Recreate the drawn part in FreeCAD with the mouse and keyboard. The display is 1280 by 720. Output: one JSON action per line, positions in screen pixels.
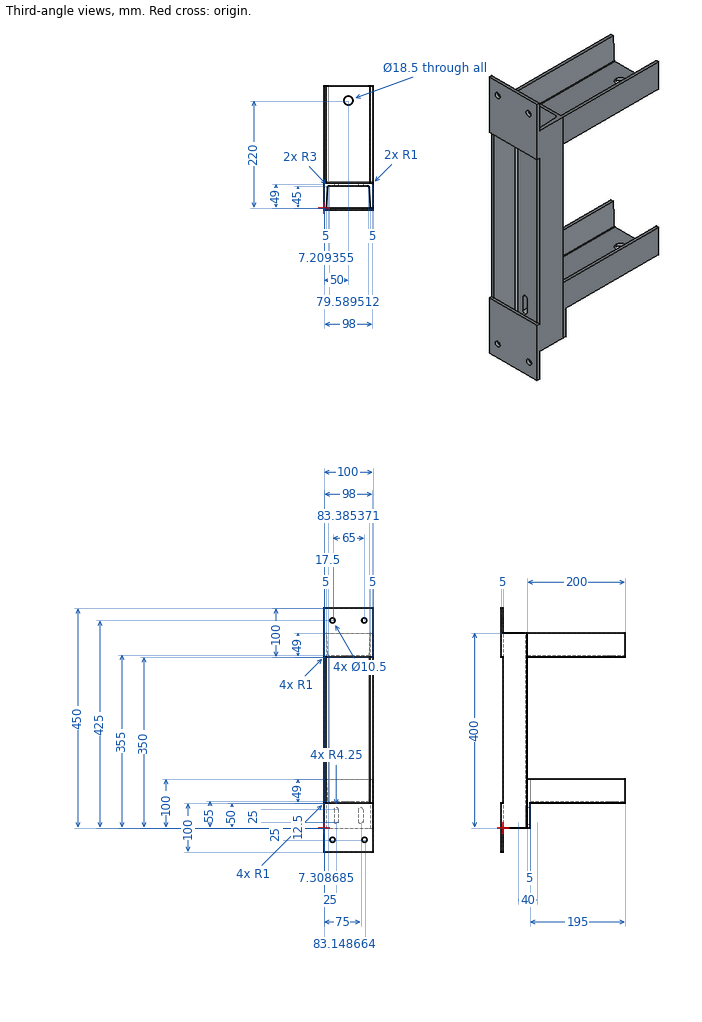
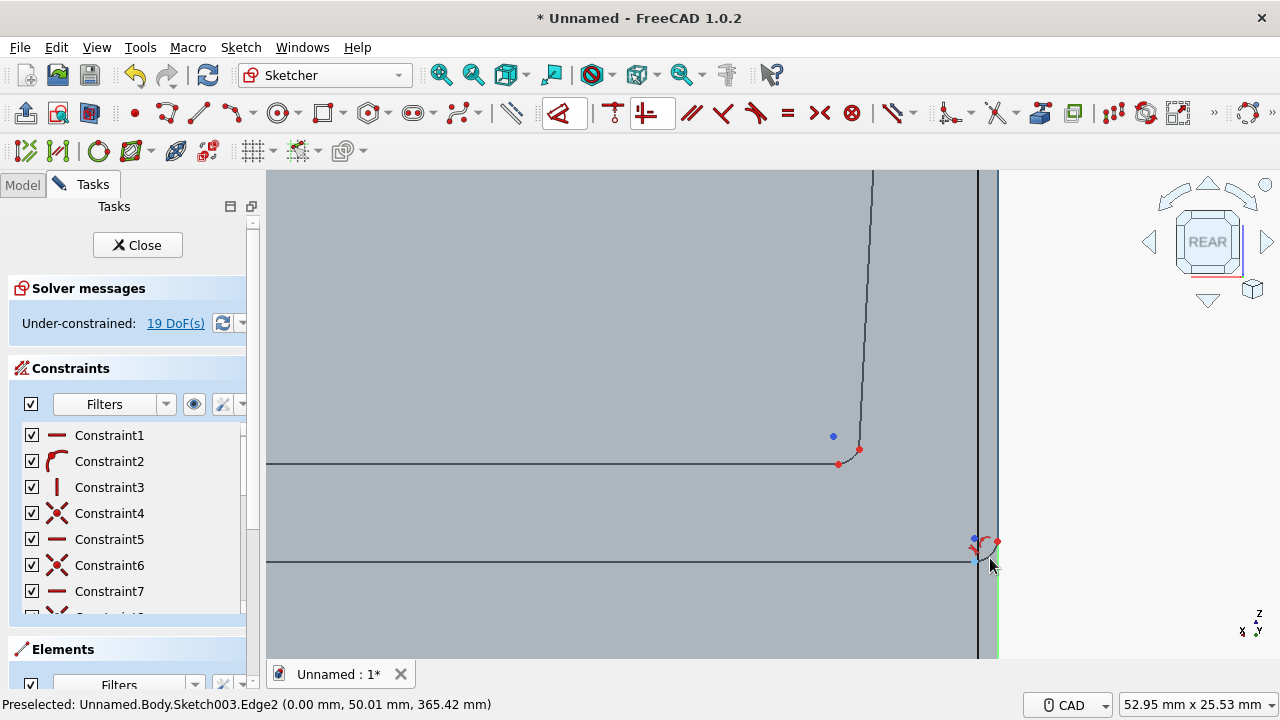
{"action": "left_click", "coordinate": [990, 556]}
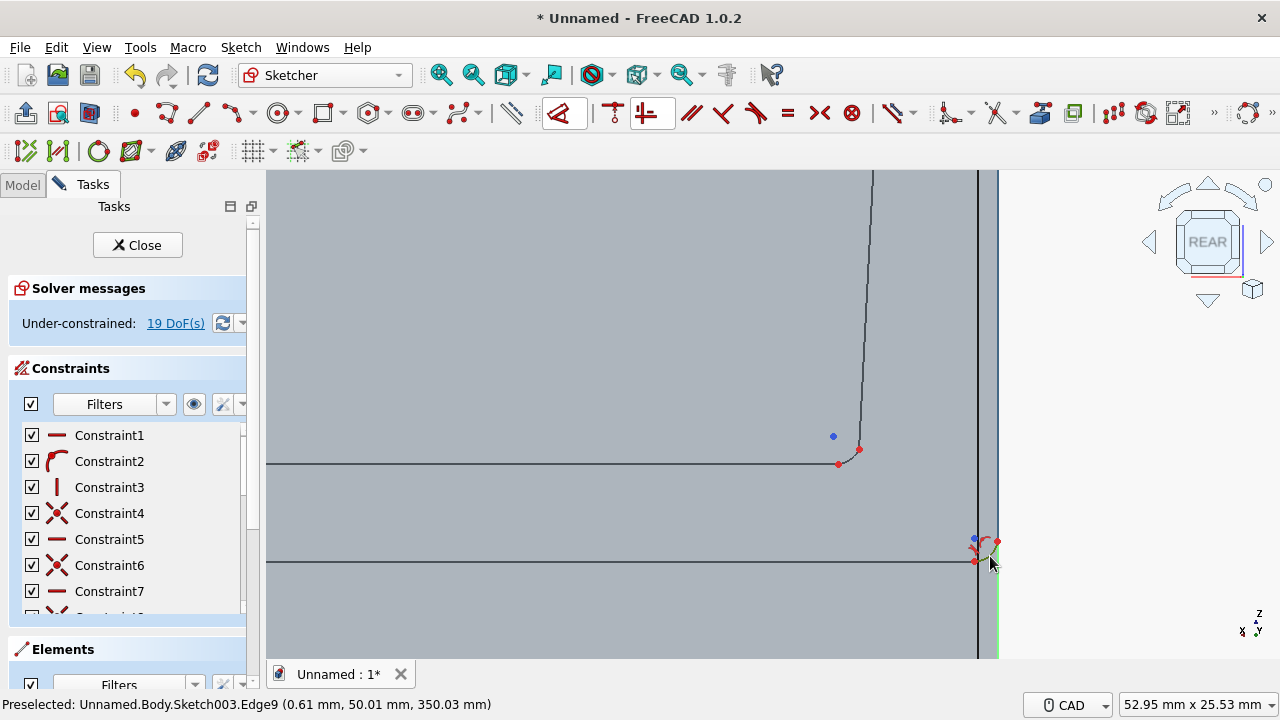
{"action": "left_click", "coordinate": [756, 114]}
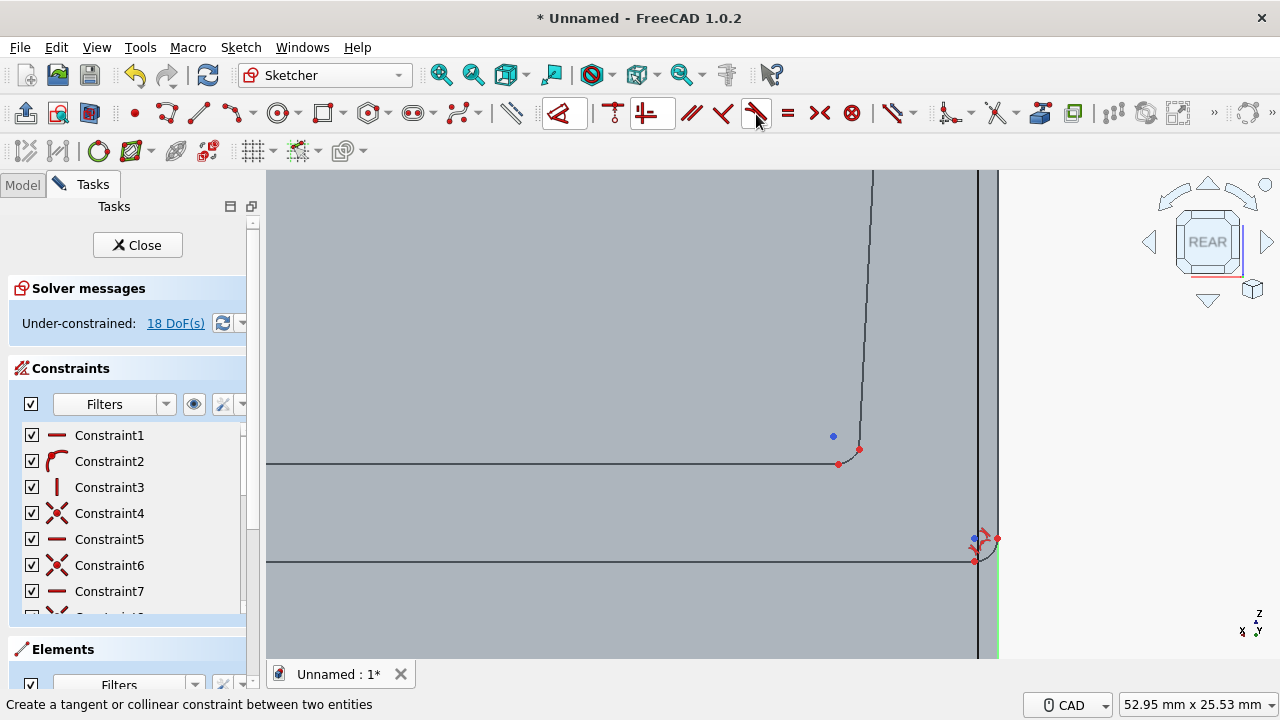
{"action": "left_click", "coordinate": [868, 281]}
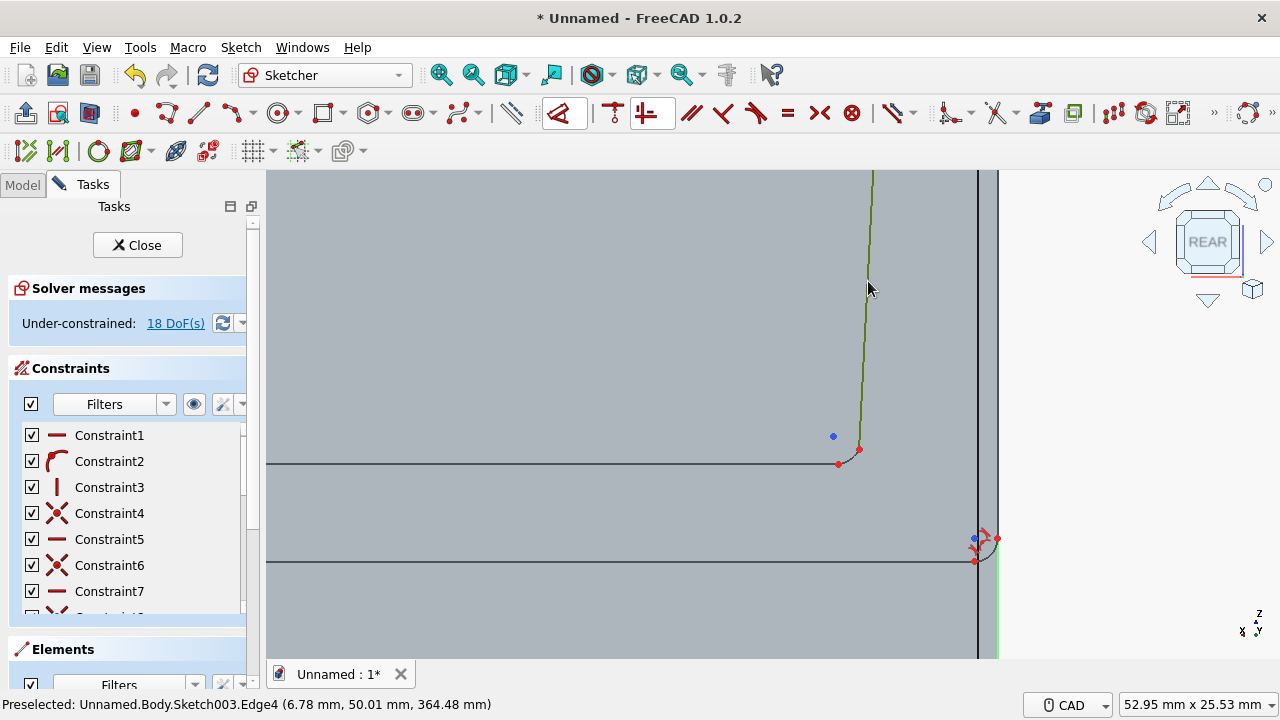
{"action": "left_click", "coordinate": [851, 459]}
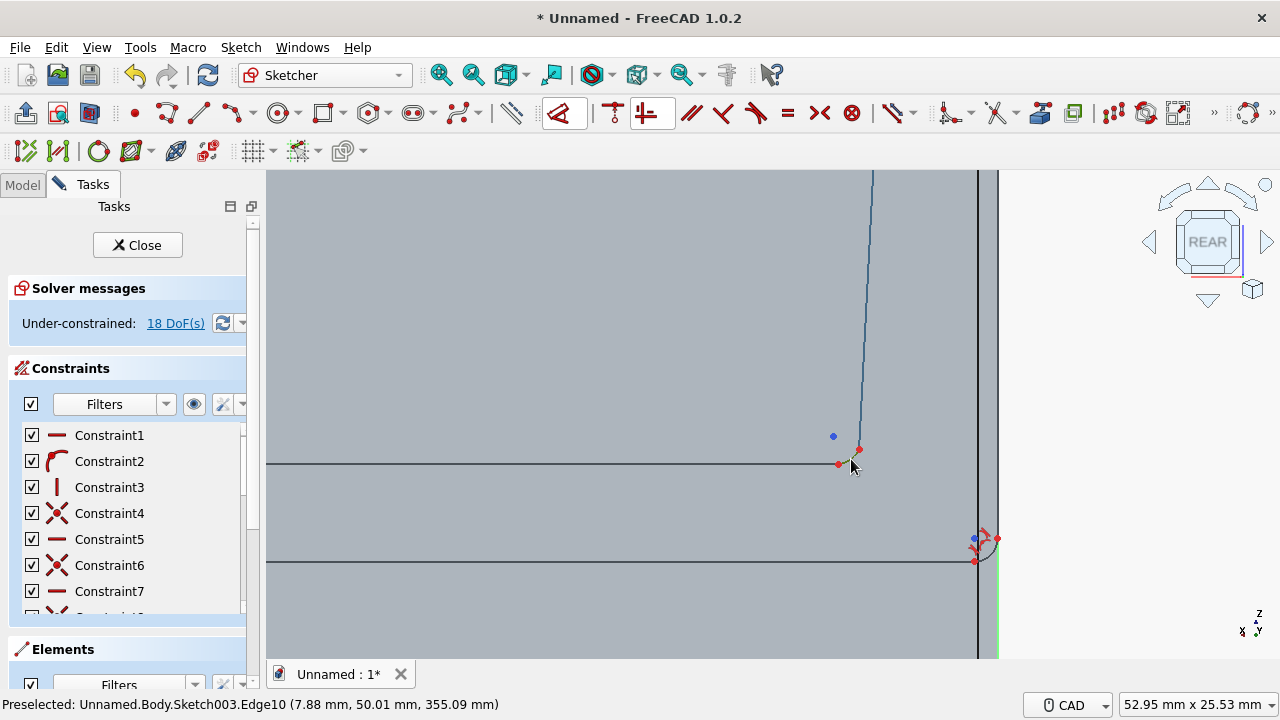
{"action": "left_click", "coordinate": [756, 114]}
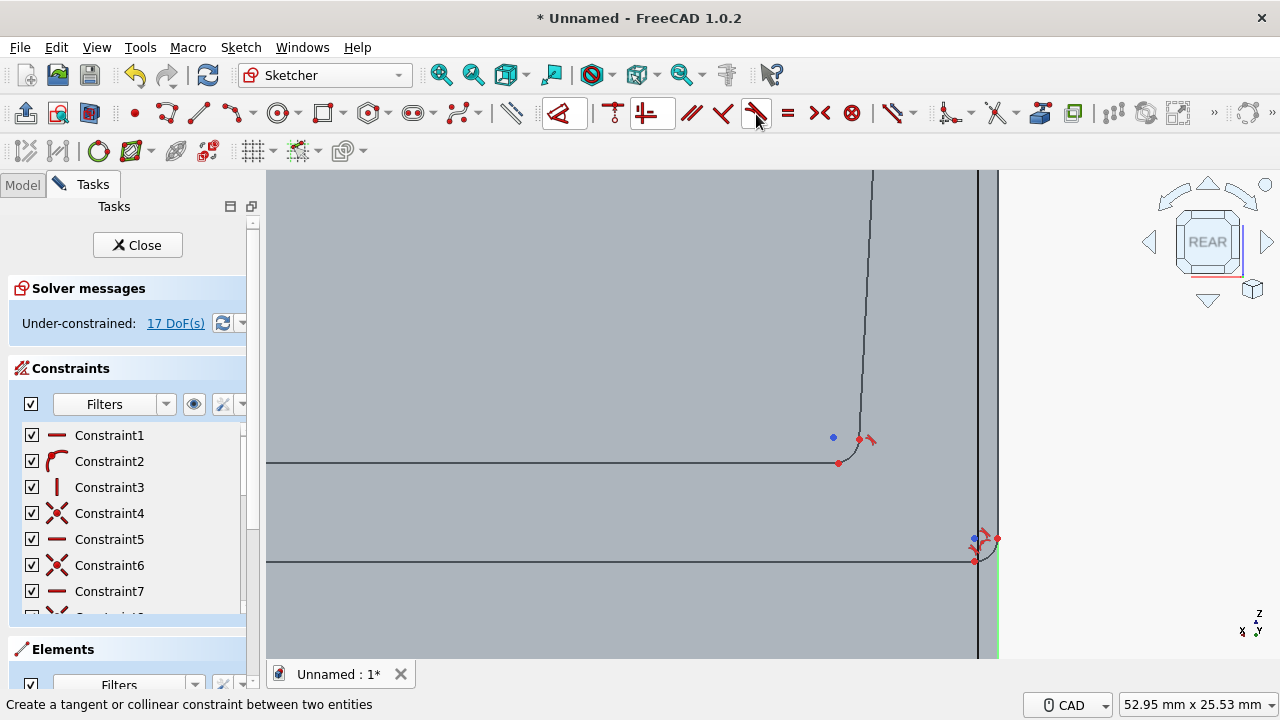
{"action": "left_click", "coordinate": [359, 463]}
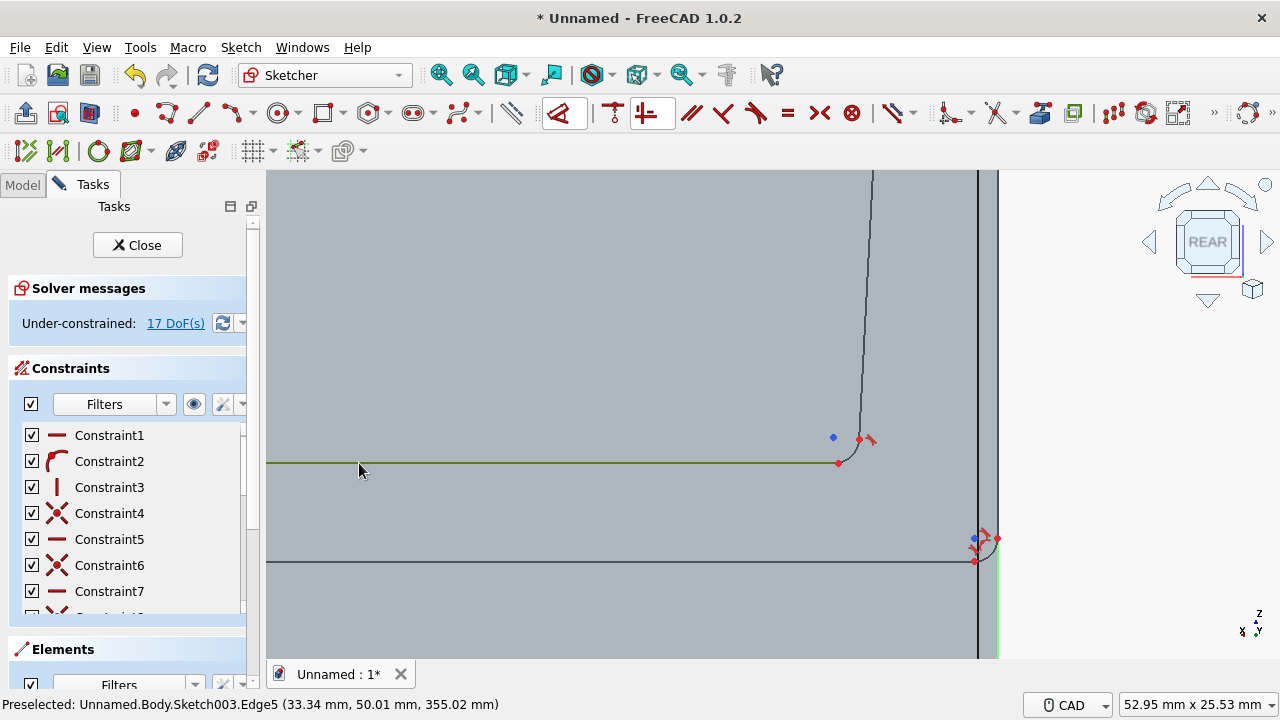
{"action": "scroll", "coordinate": [848, 459], "scroll_direction": "up", "scroll_amount": 2}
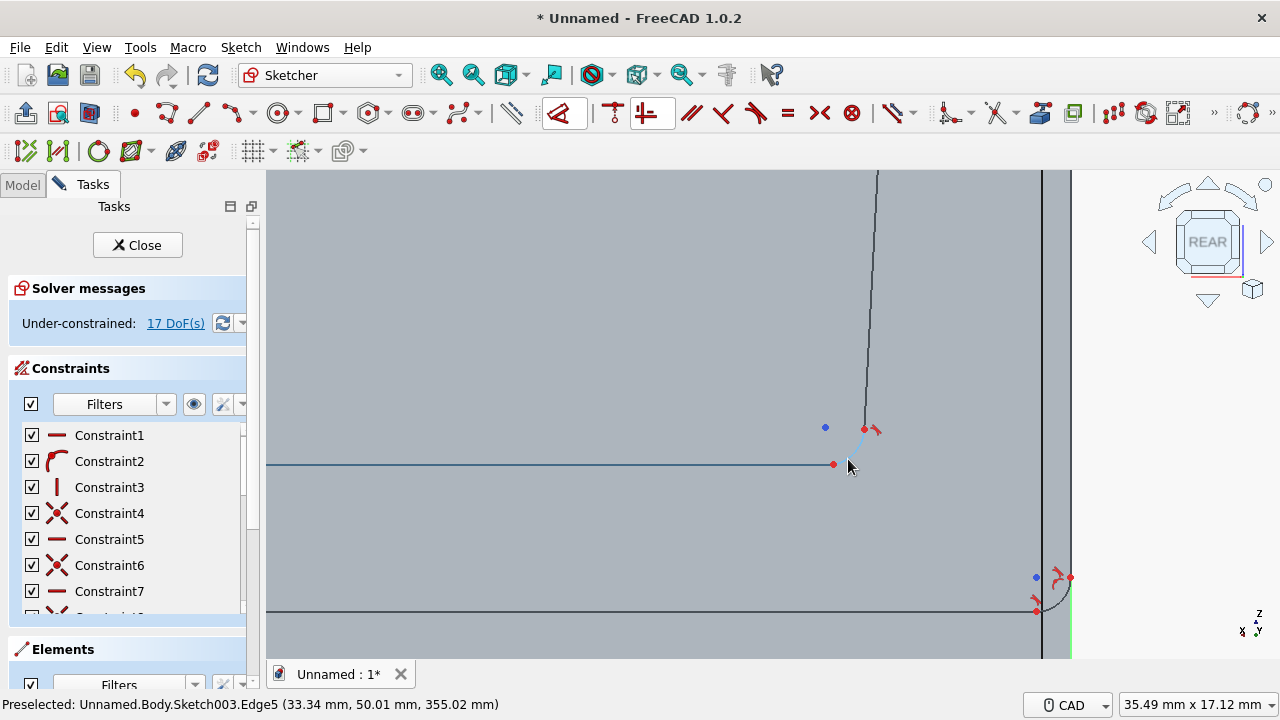
{"action": "left_click", "coordinate": [847, 459]}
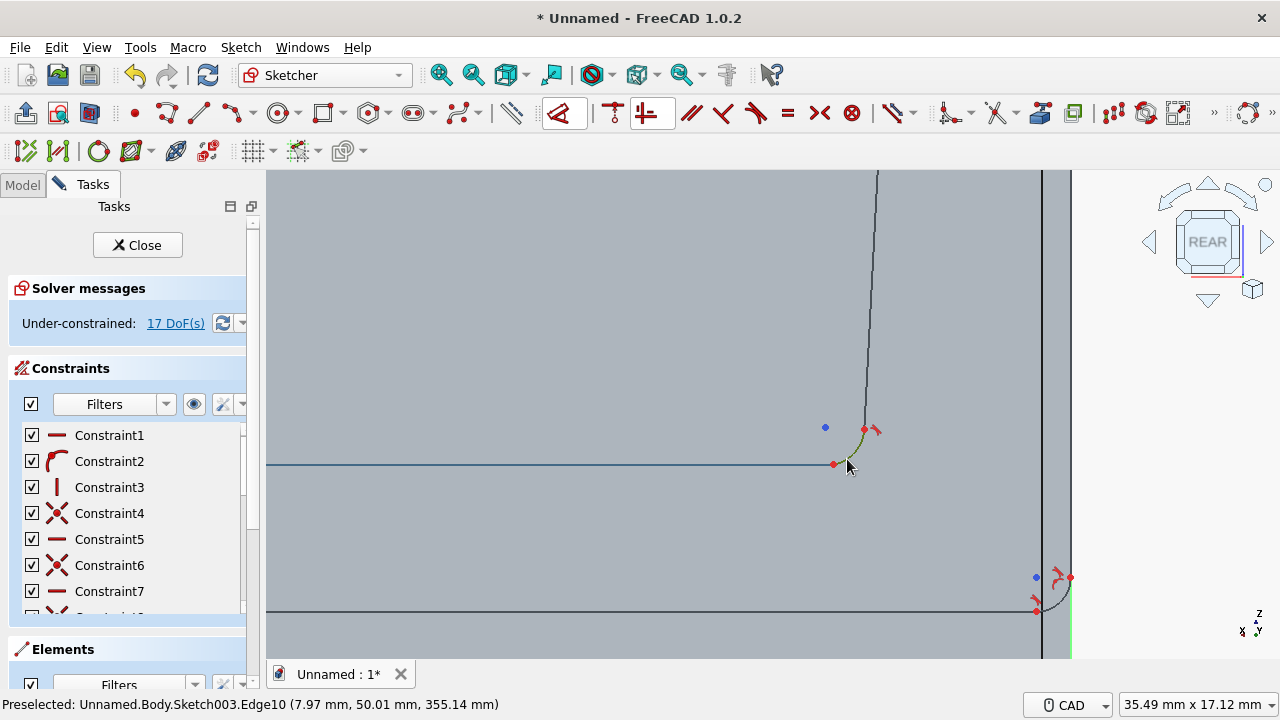
{"action": "left_click", "coordinate": [756, 114]}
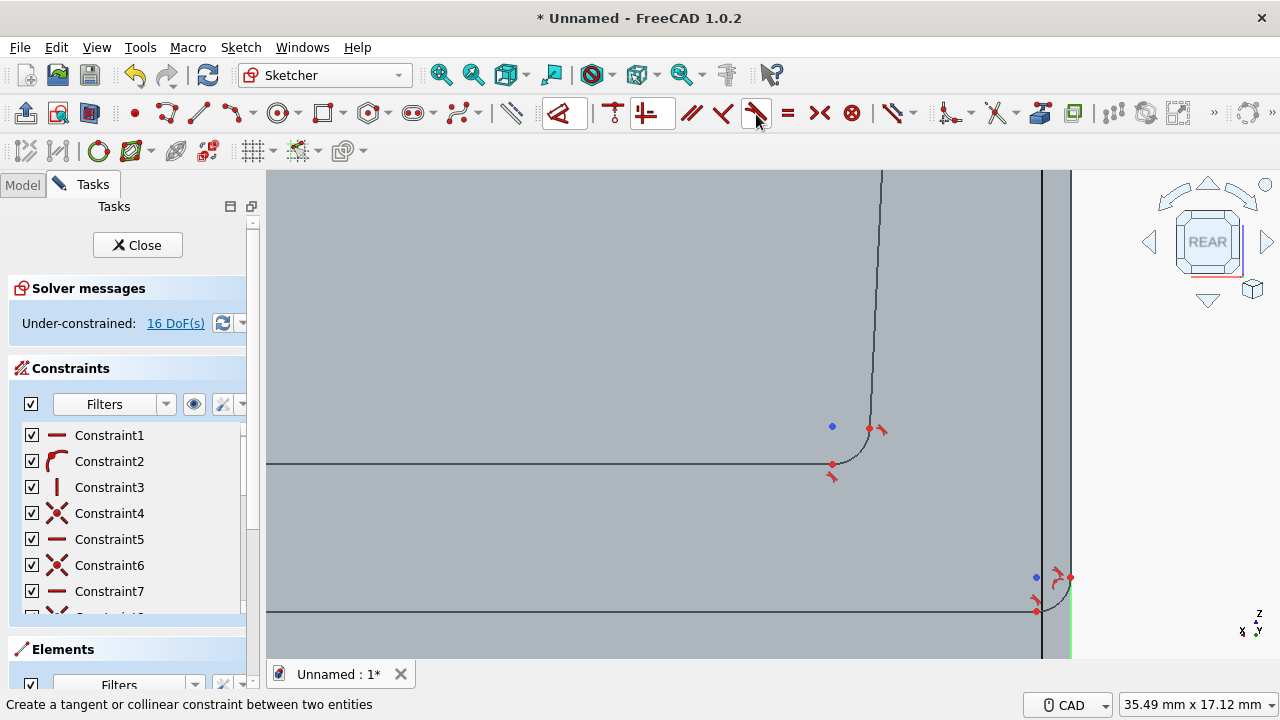
{"action": "scroll", "coordinate": [973, 546], "scroll_direction": "down", "scroll_amount": 8}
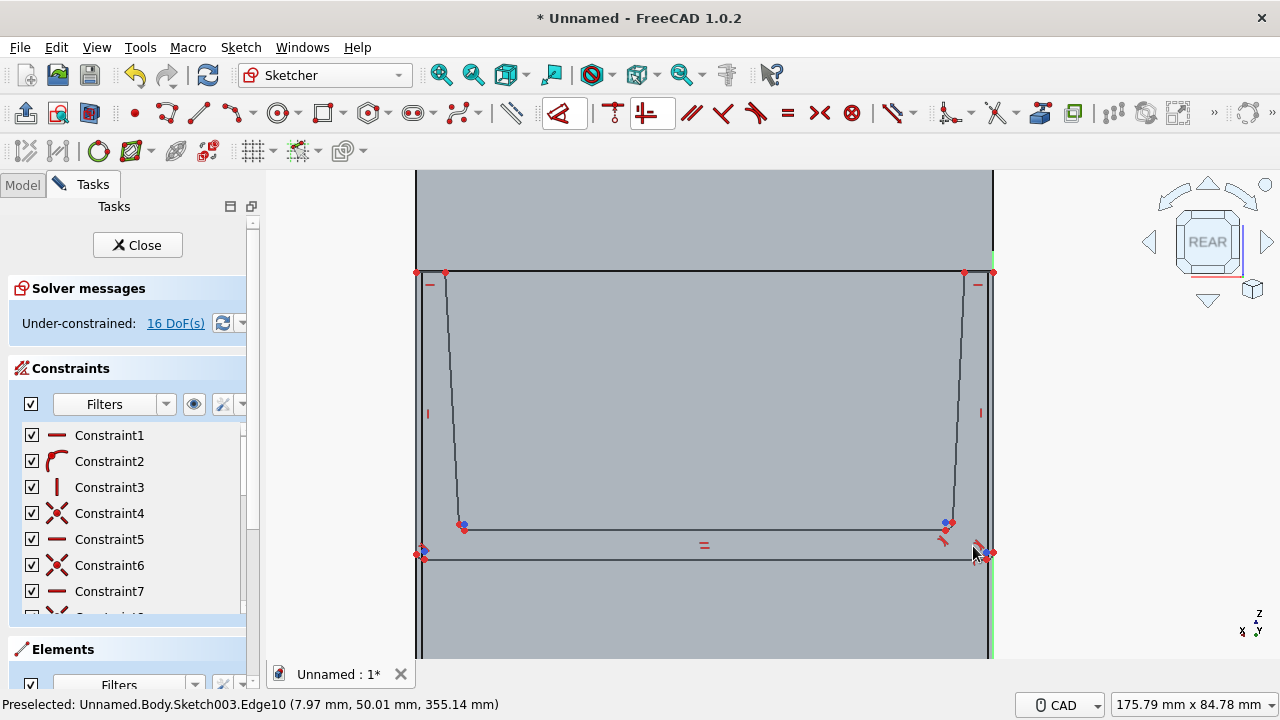
{"action": "left_click", "coordinate": [849, 530]}